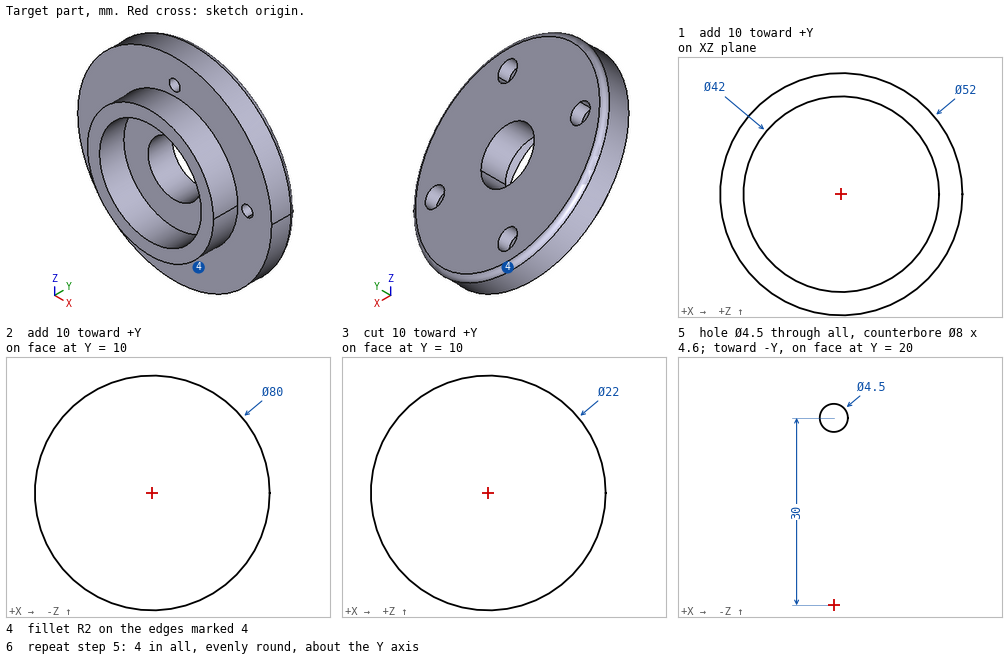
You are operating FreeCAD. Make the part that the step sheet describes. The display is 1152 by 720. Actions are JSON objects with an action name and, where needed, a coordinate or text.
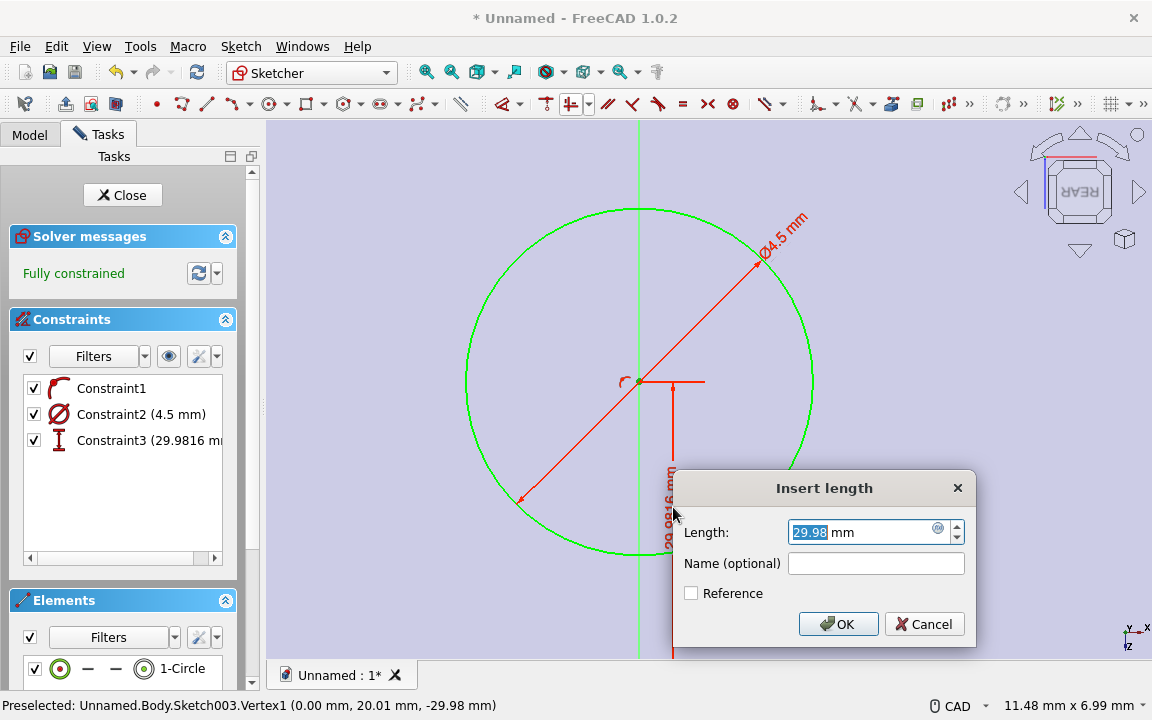
{"action": "type", "text": "30"}
{"action": "key", "text": "Return"}
{"action": "key", "text": "Escape"}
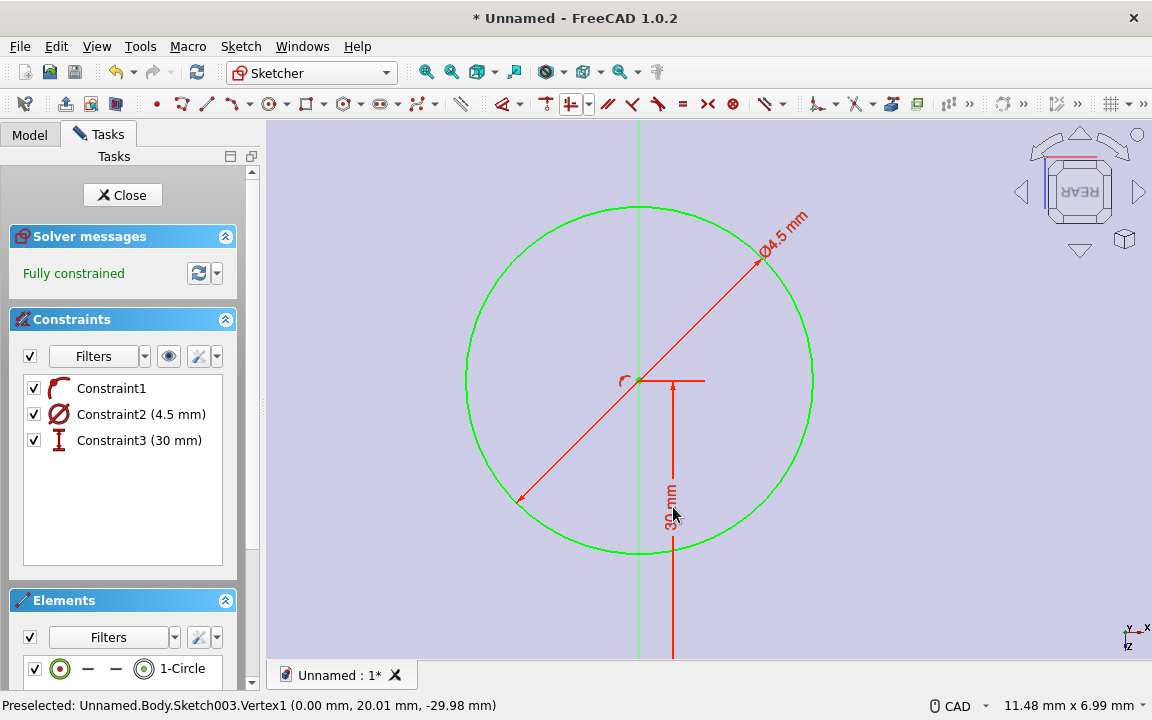
{"action": "left_click", "coordinate": [123, 195]}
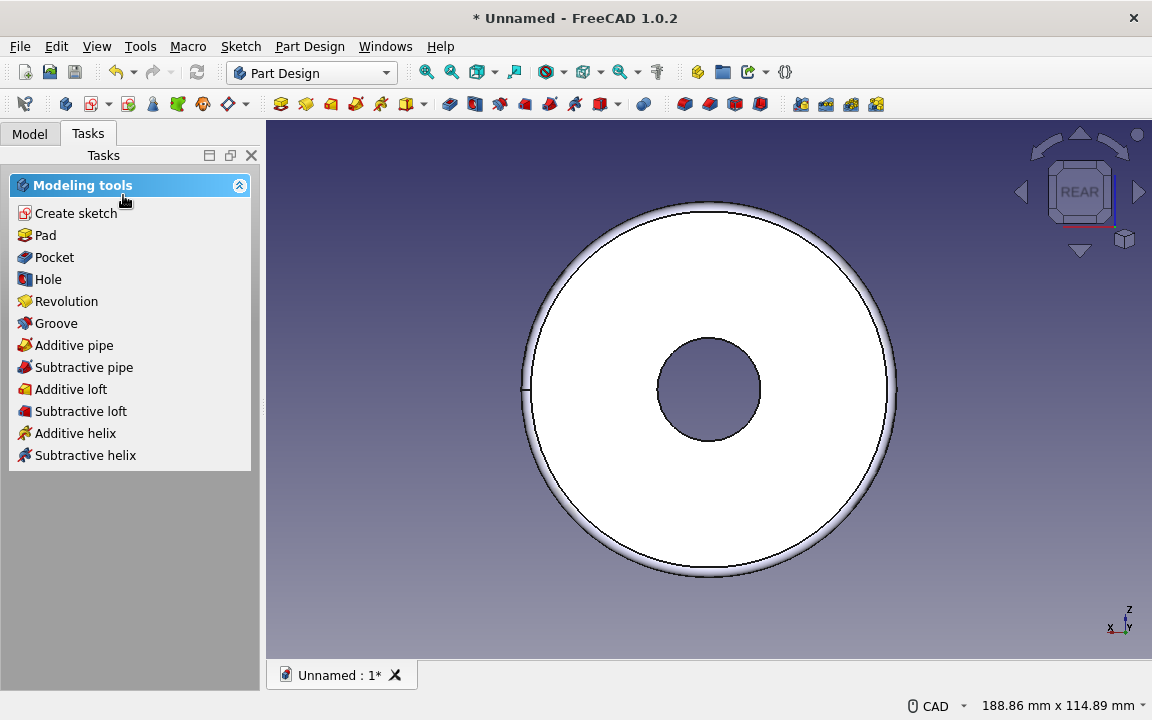
{"action": "left_click", "coordinate": [475, 104]}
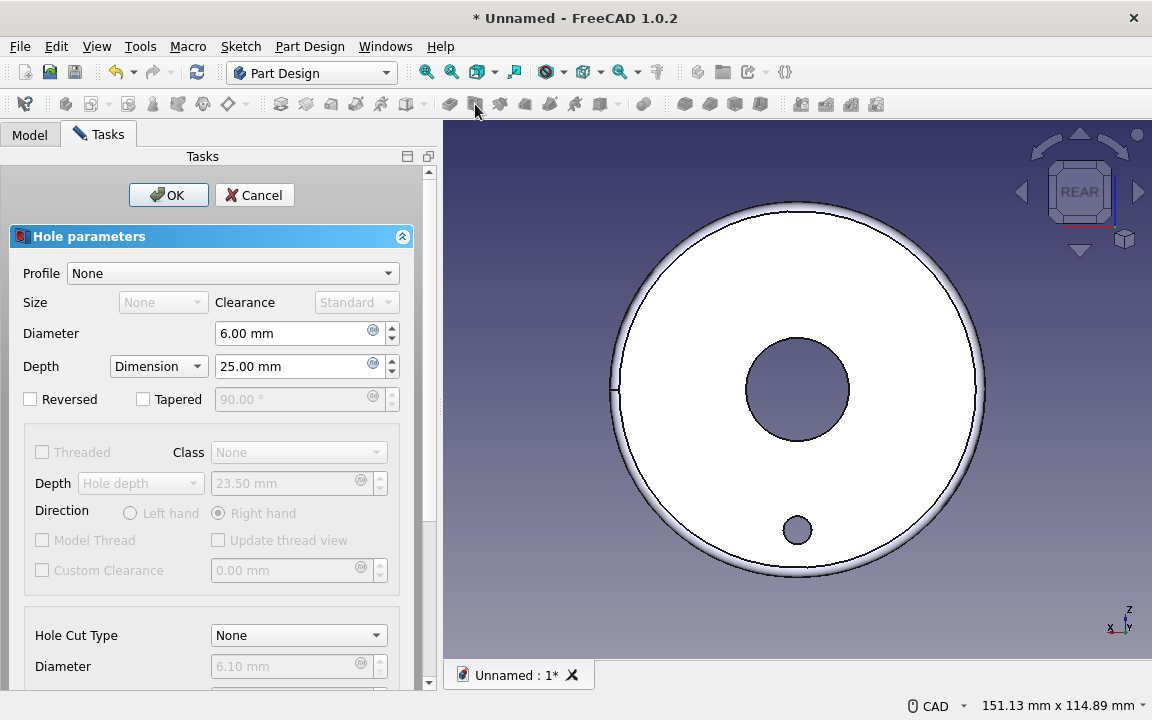
{"action": "triple_click", "coordinate": [300, 334]}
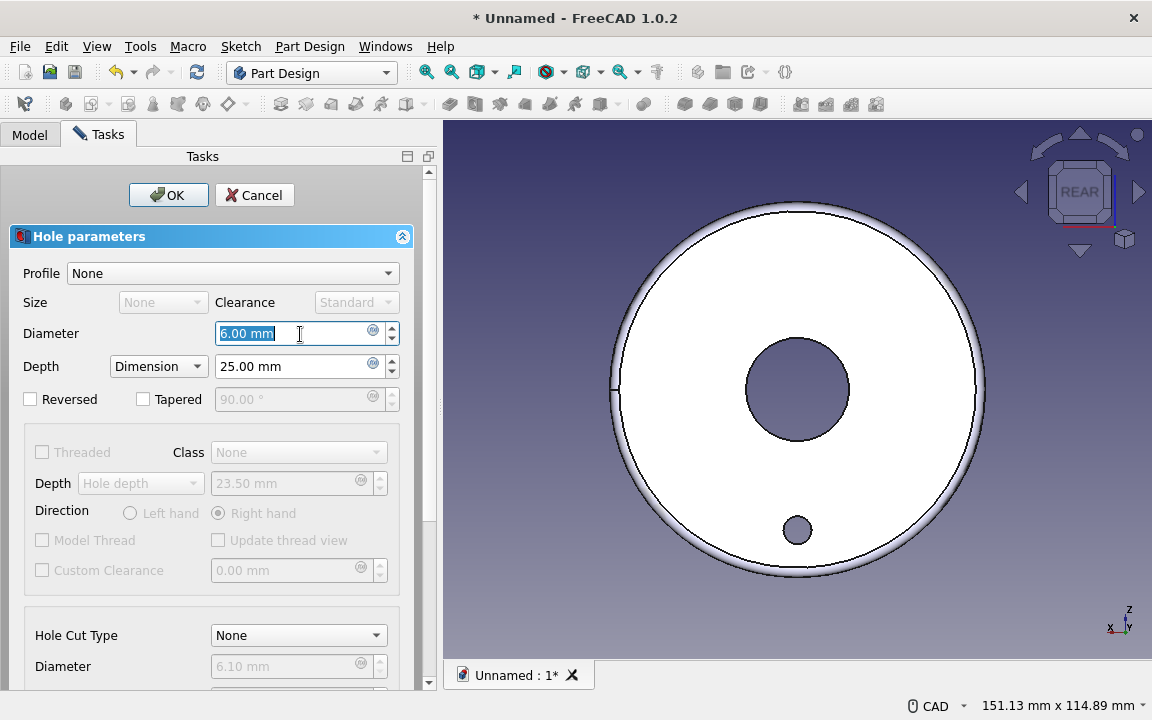
{"action": "type", "text": "4.5"}
{"action": "key", "text": "Tab"}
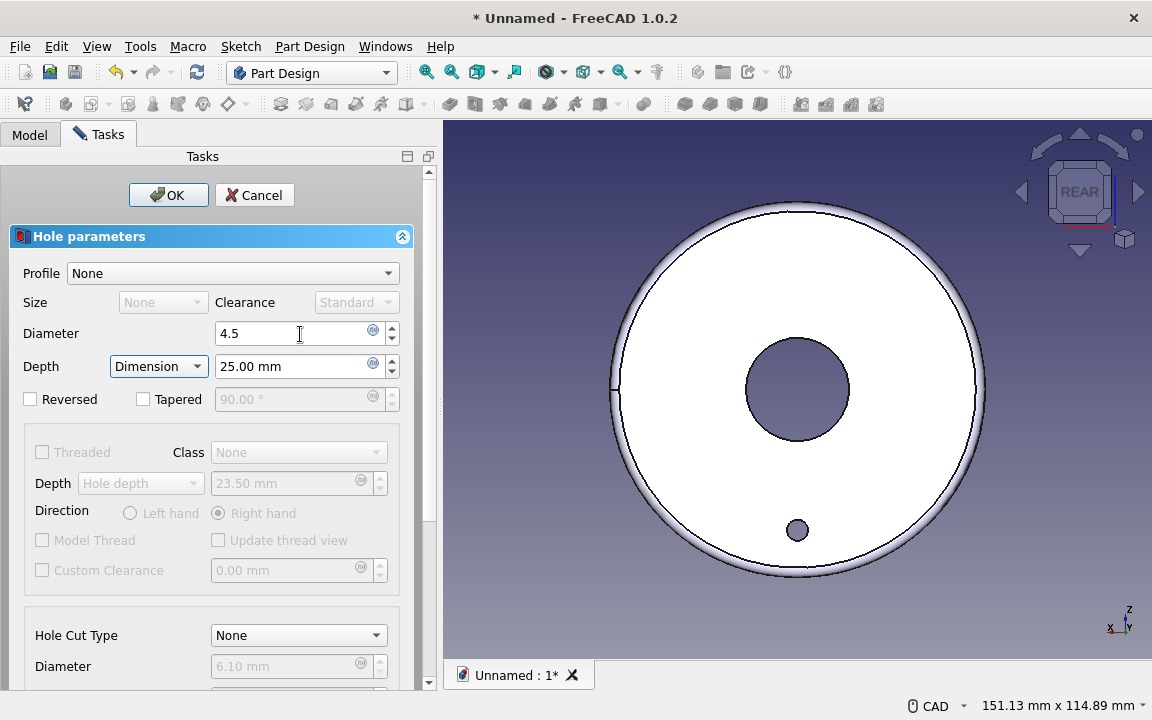
{"action": "left_click", "coordinate": [160, 366]}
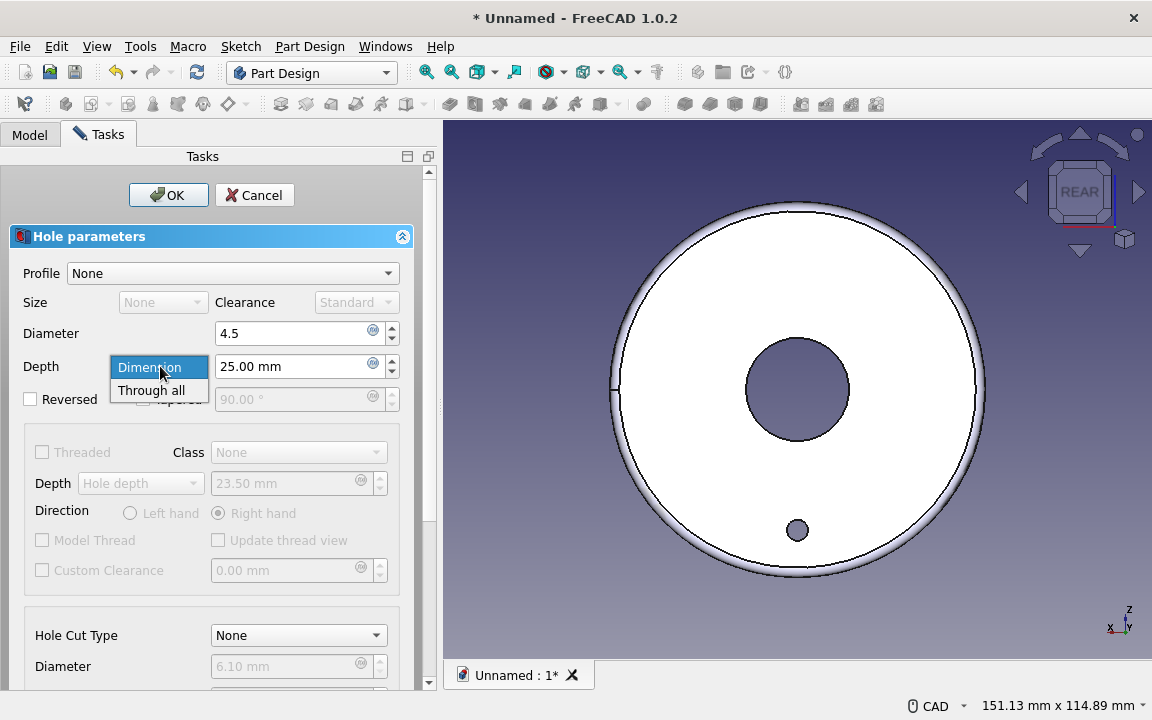
{"action": "left_click", "coordinate": [158, 390]}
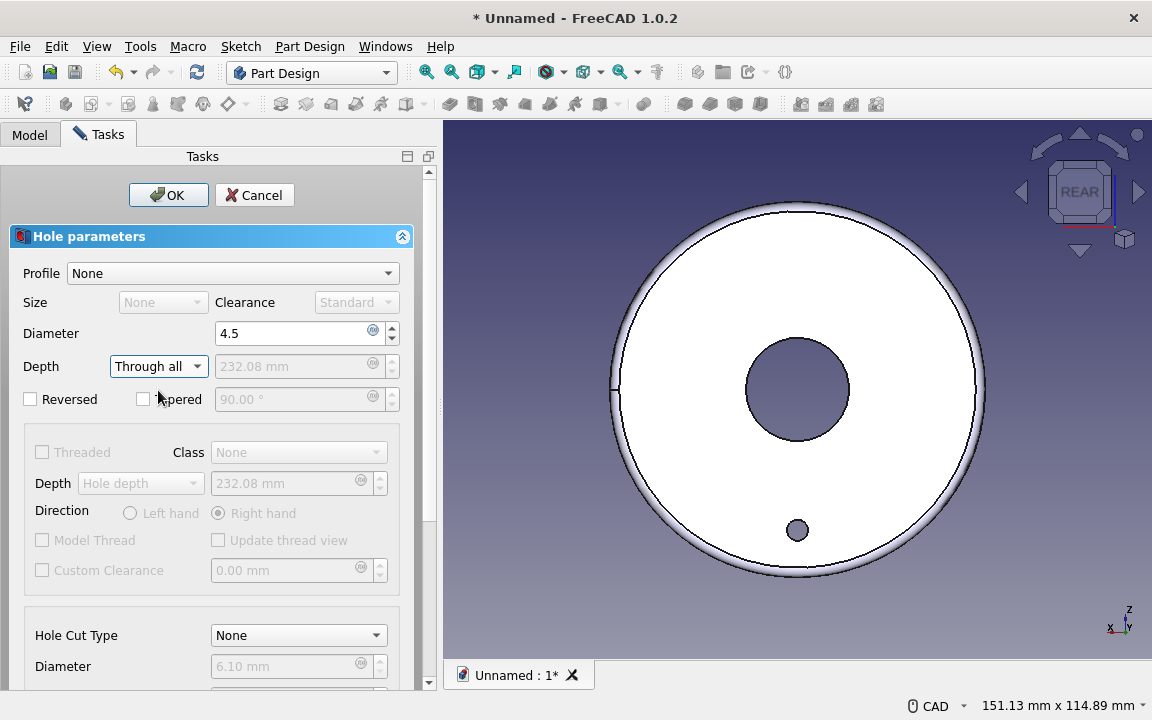
{"action": "left_click", "coordinate": [300, 636]}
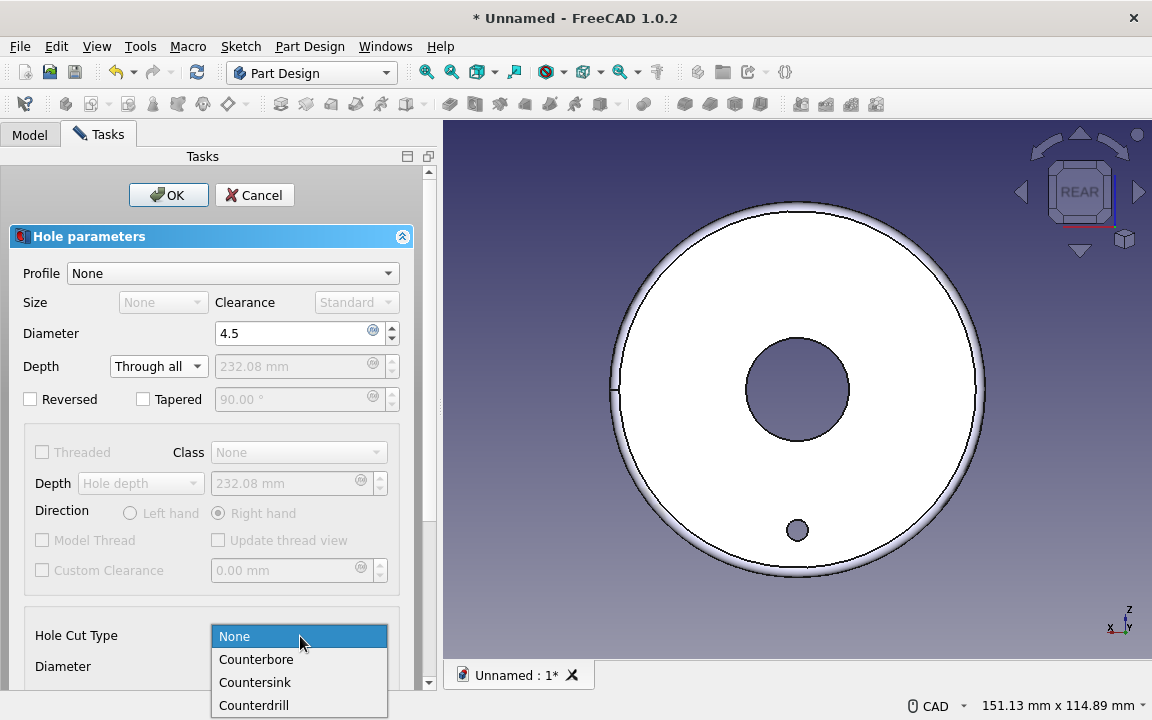
{"action": "left_click", "coordinate": [298, 660]}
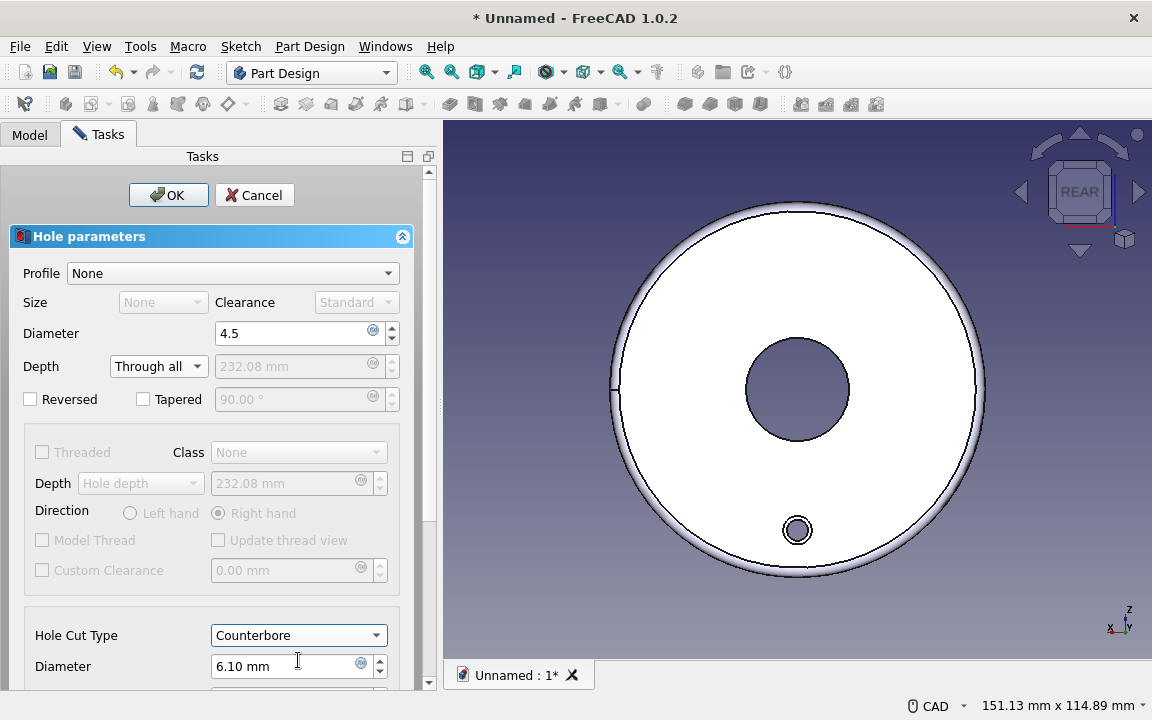
{"action": "triple_click", "coordinate": [292, 666]}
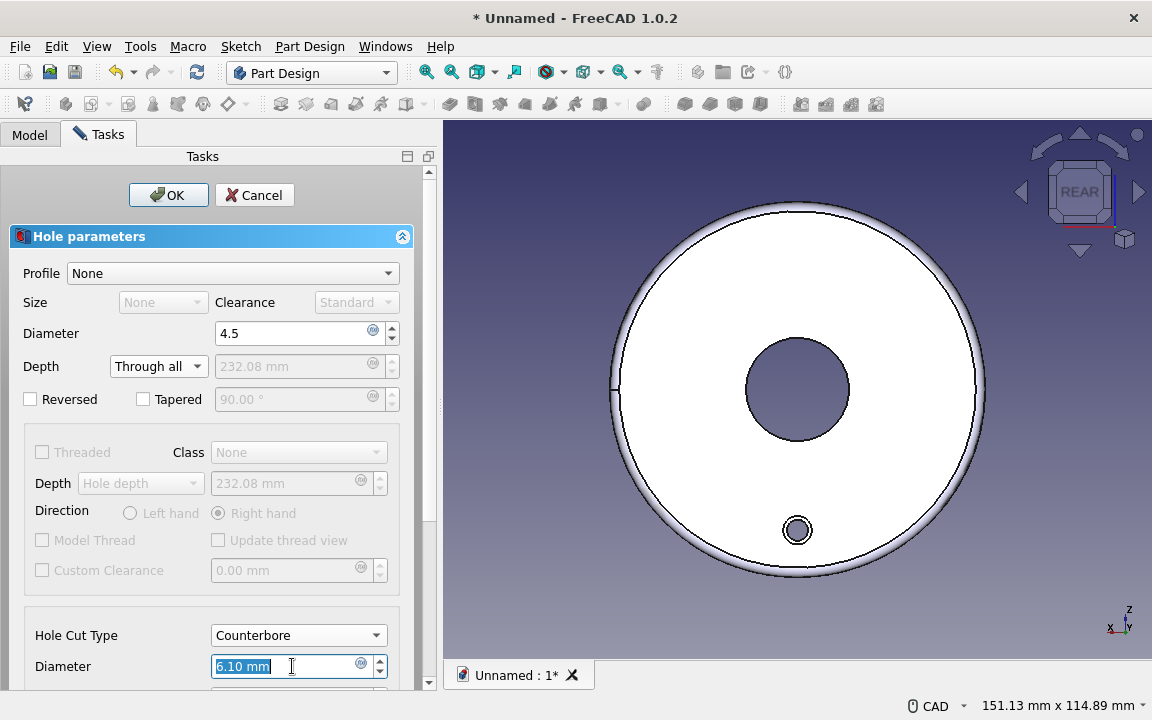
{"action": "type", "text": "8"}
{"action": "key", "text": "Tab"}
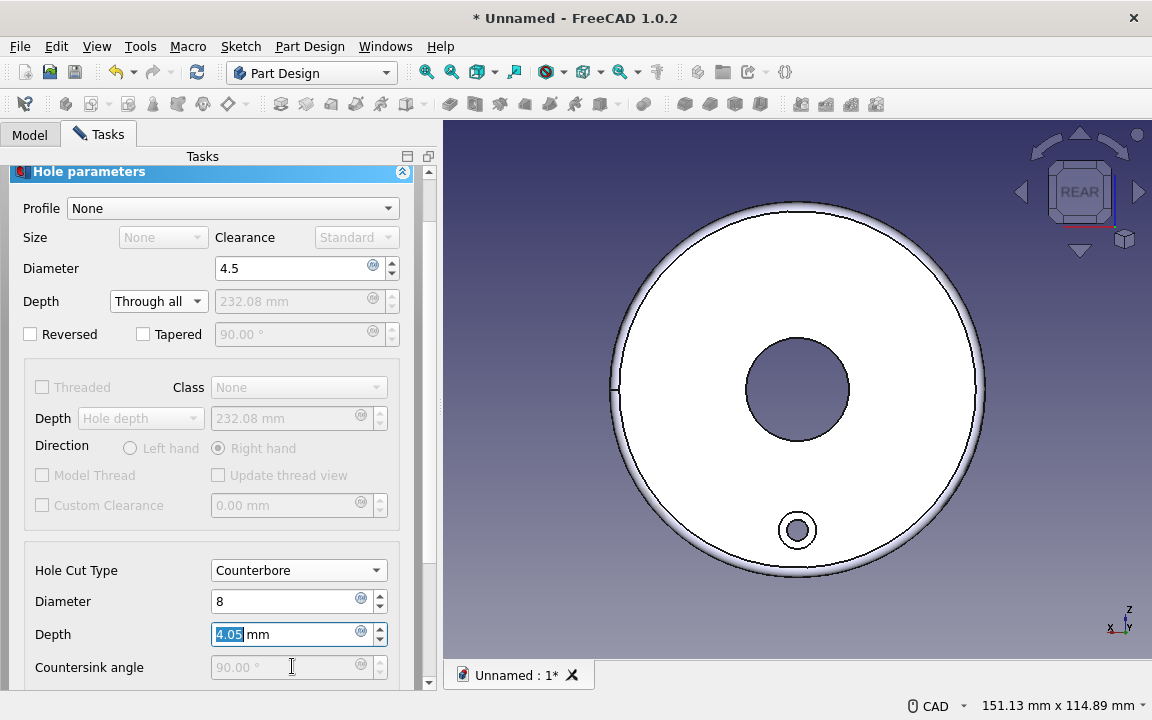
{"action": "type", "text": "4.6"}
{"action": "key", "text": "Tab"}